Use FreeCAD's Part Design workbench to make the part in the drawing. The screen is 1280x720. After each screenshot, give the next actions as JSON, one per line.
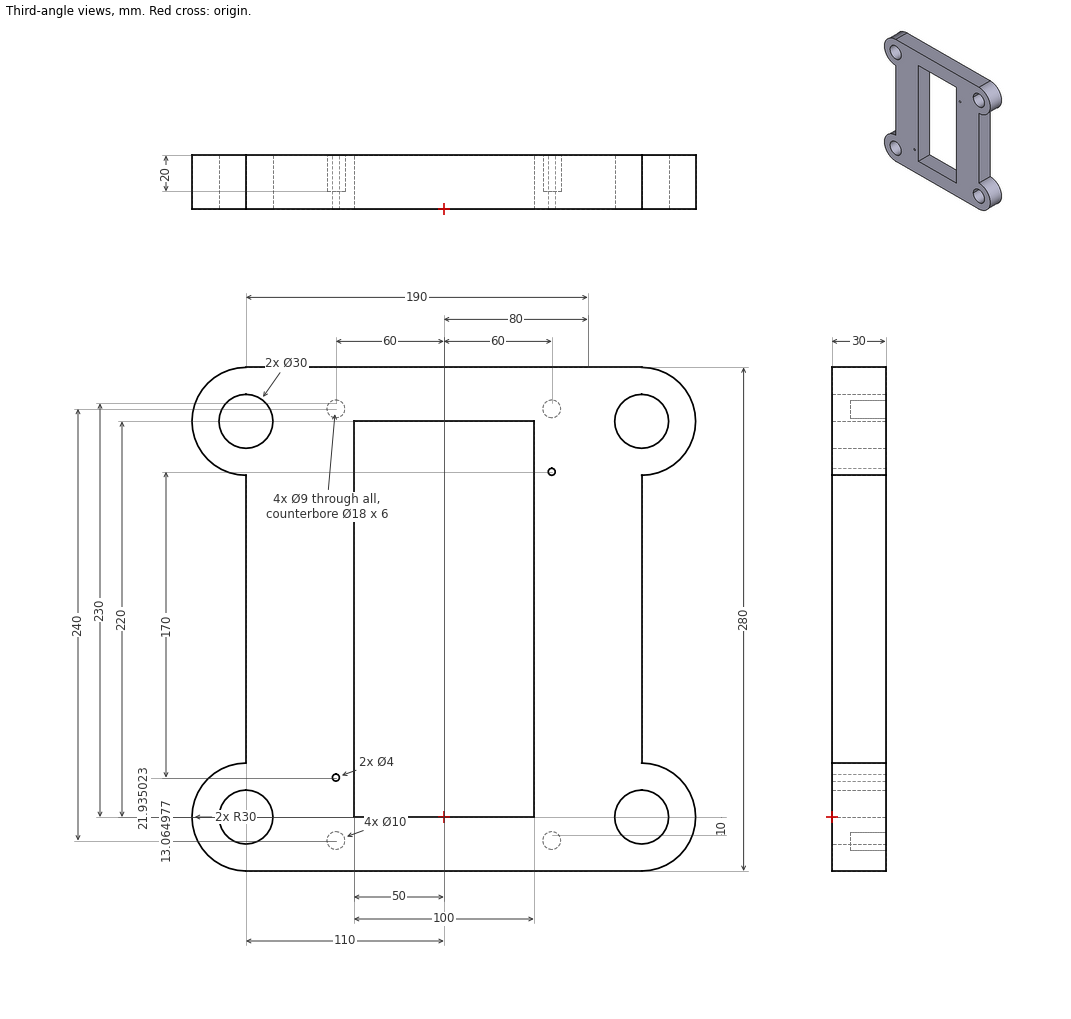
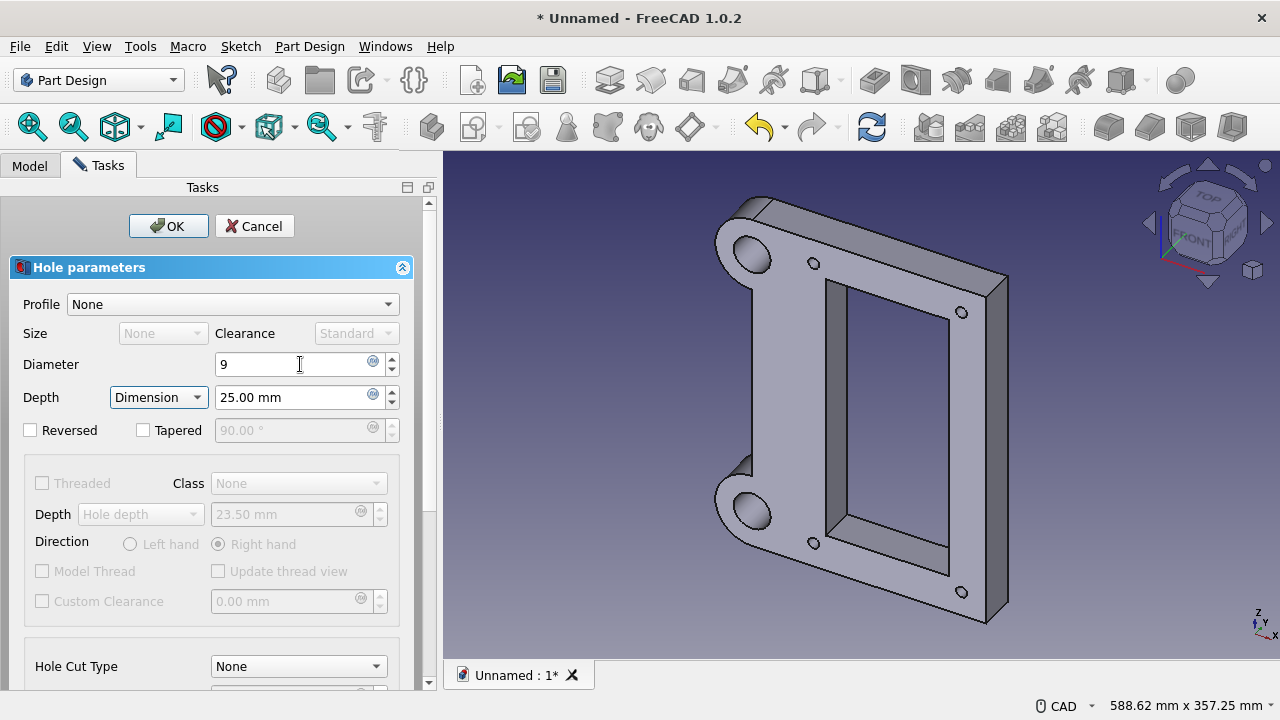
{"action": "left_click", "coordinate": [160, 398]}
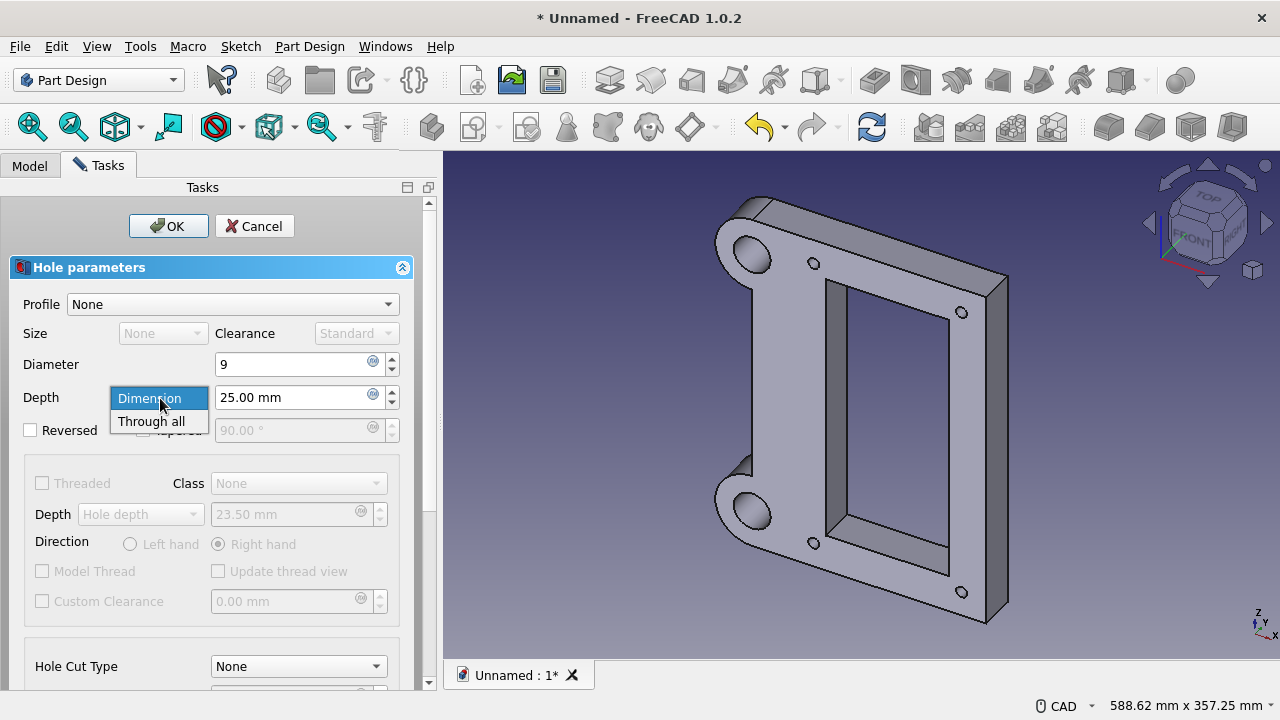
{"action": "left_click", "coordinate": [158, 422]}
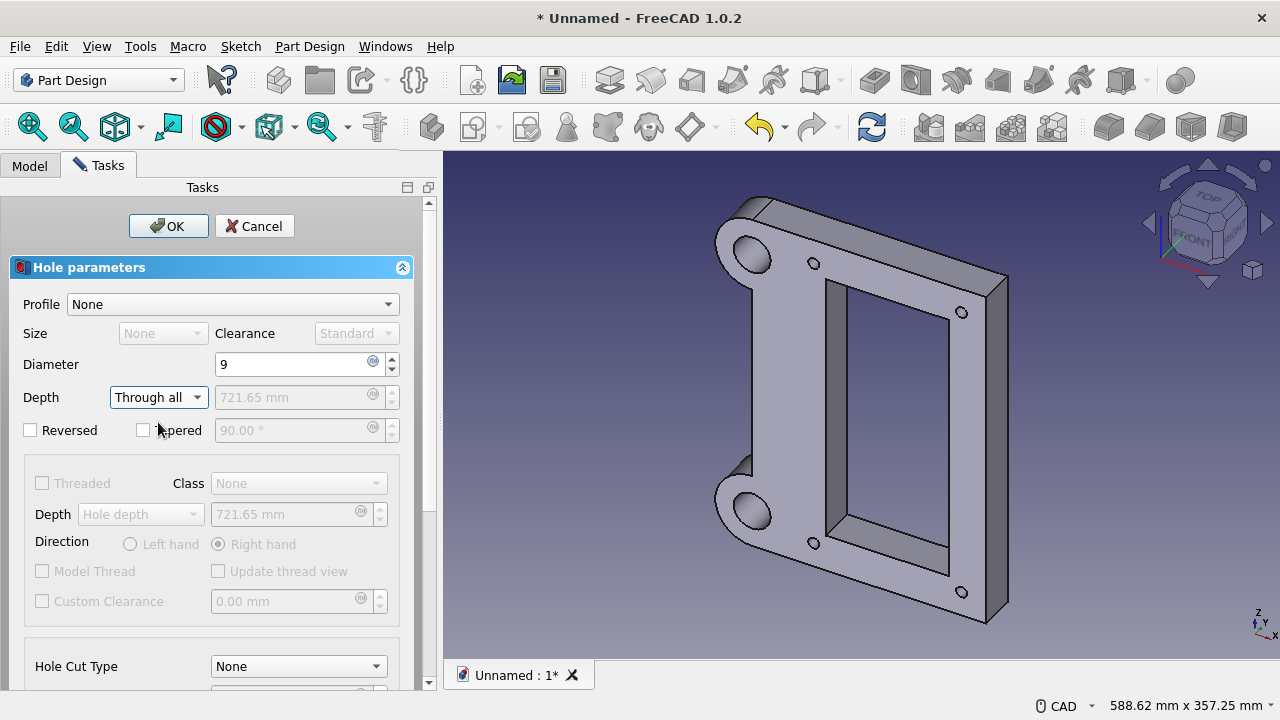
{"action": "left_click", "coordinate": [300, 666]}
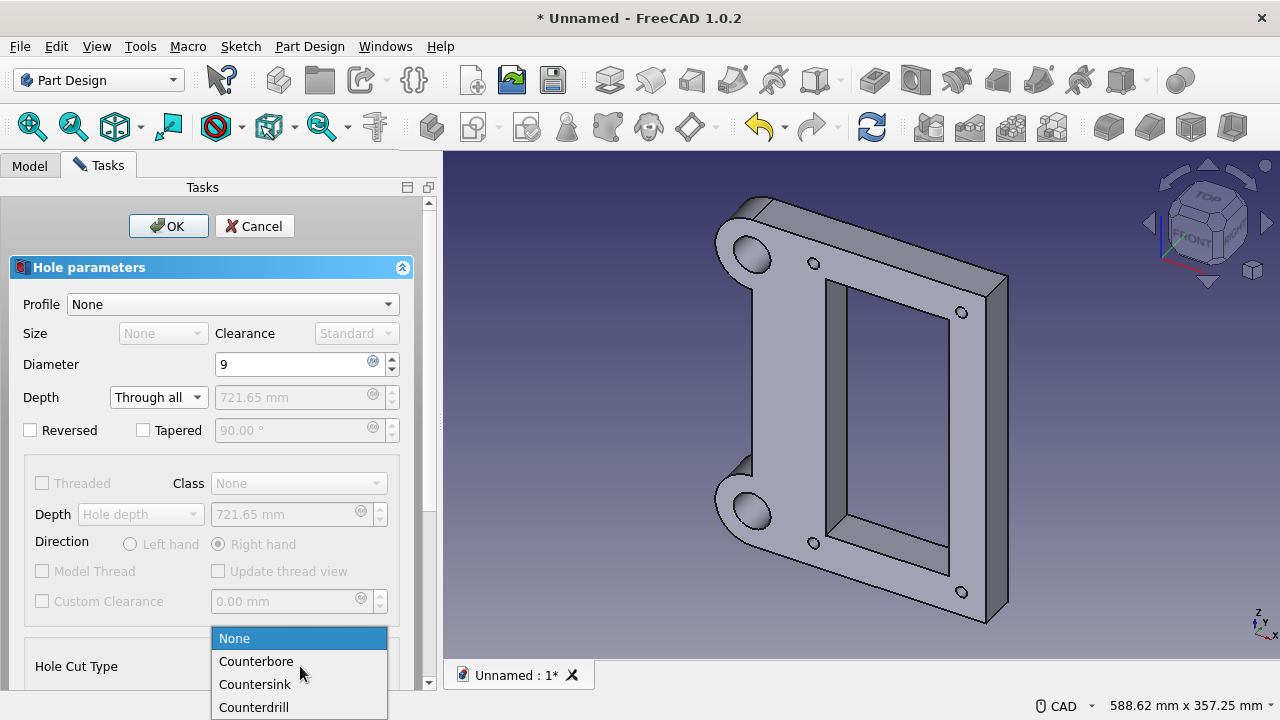
{"action": "left_click", "coordinate": [298, 662]}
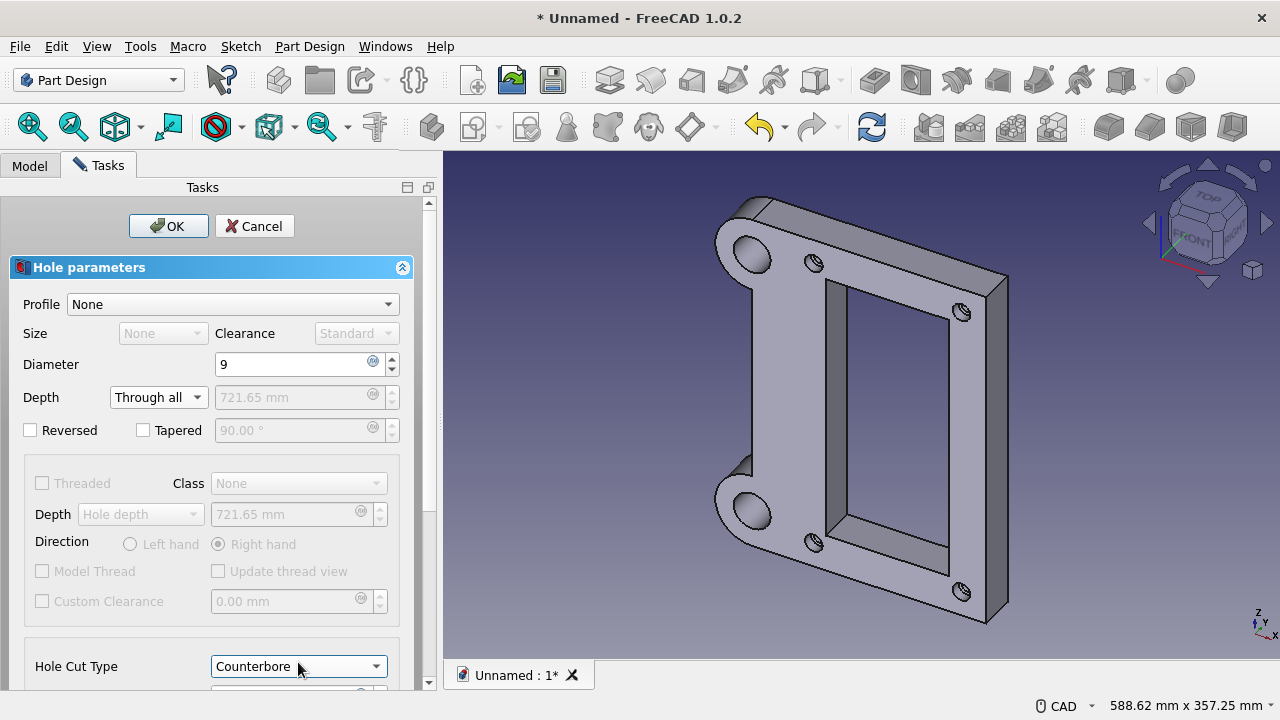
{"action": "scroll", "coordinate": [429, 444], "scroll_direction": "down", "scroll_amount": 2}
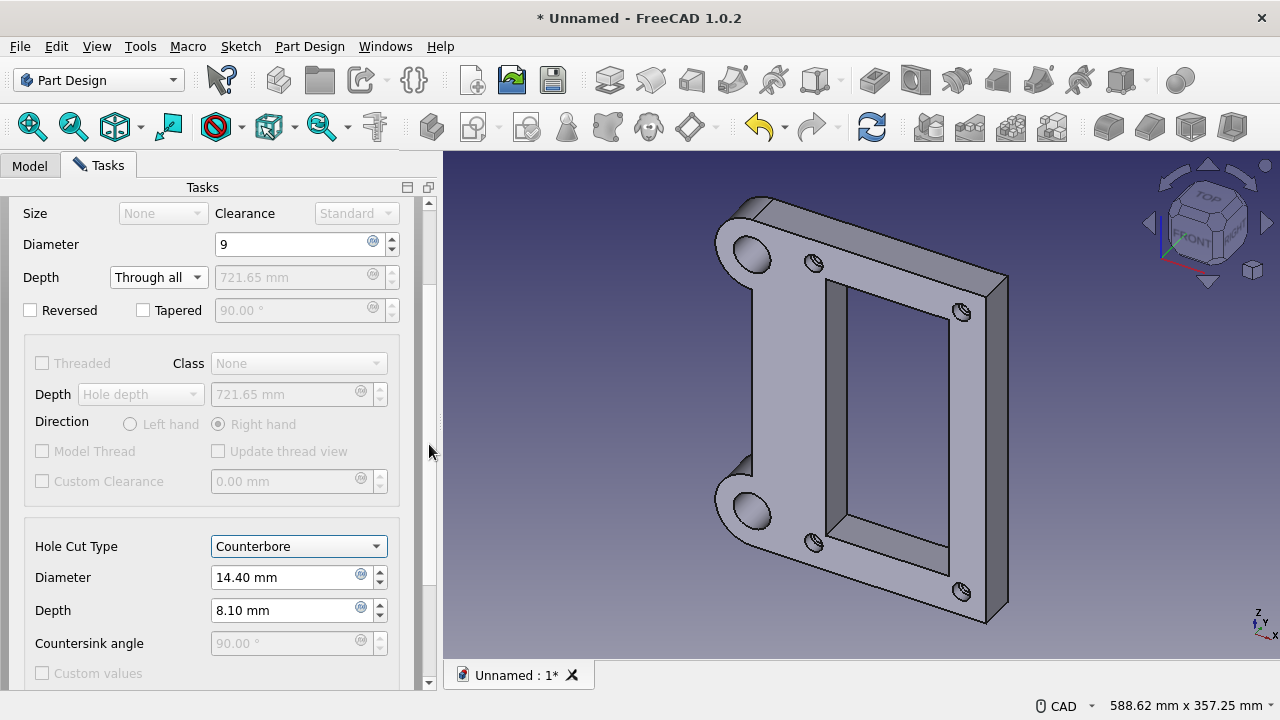
{"action": "triple_click", "coordinate": [292, 578]}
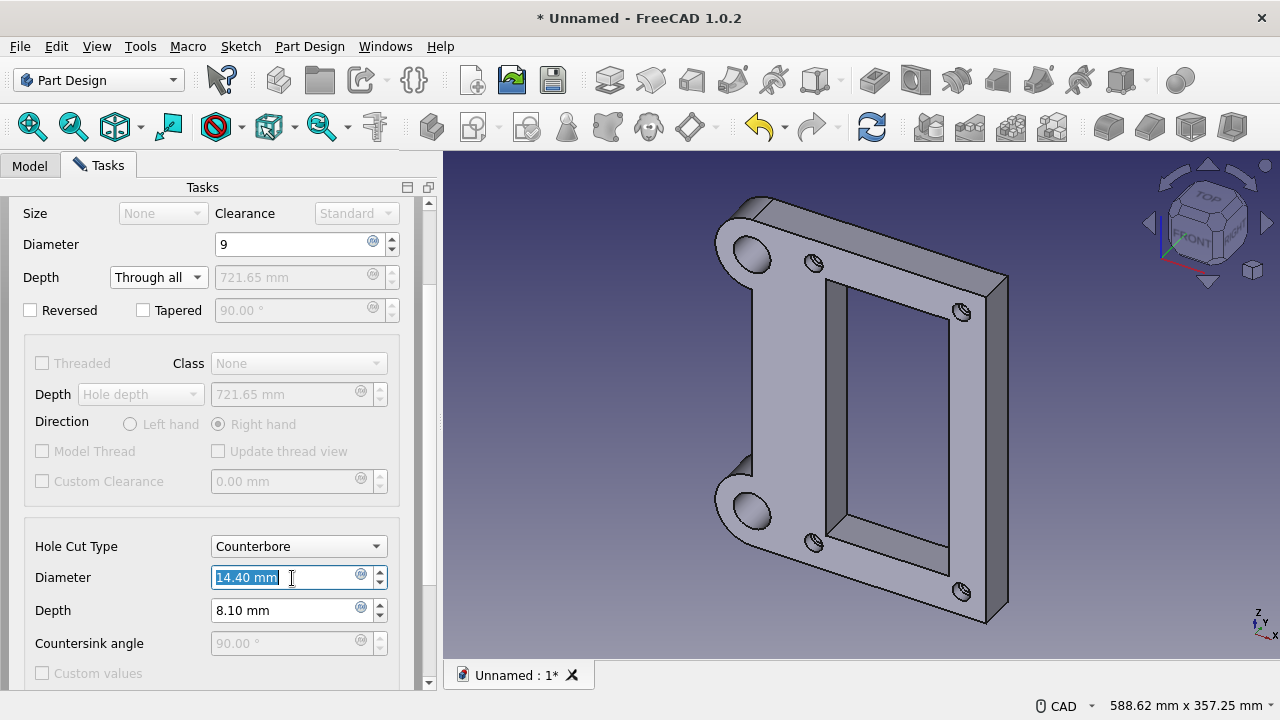
{"action": "type", "text": "18"}
{"action": "key", "text": "Tab"}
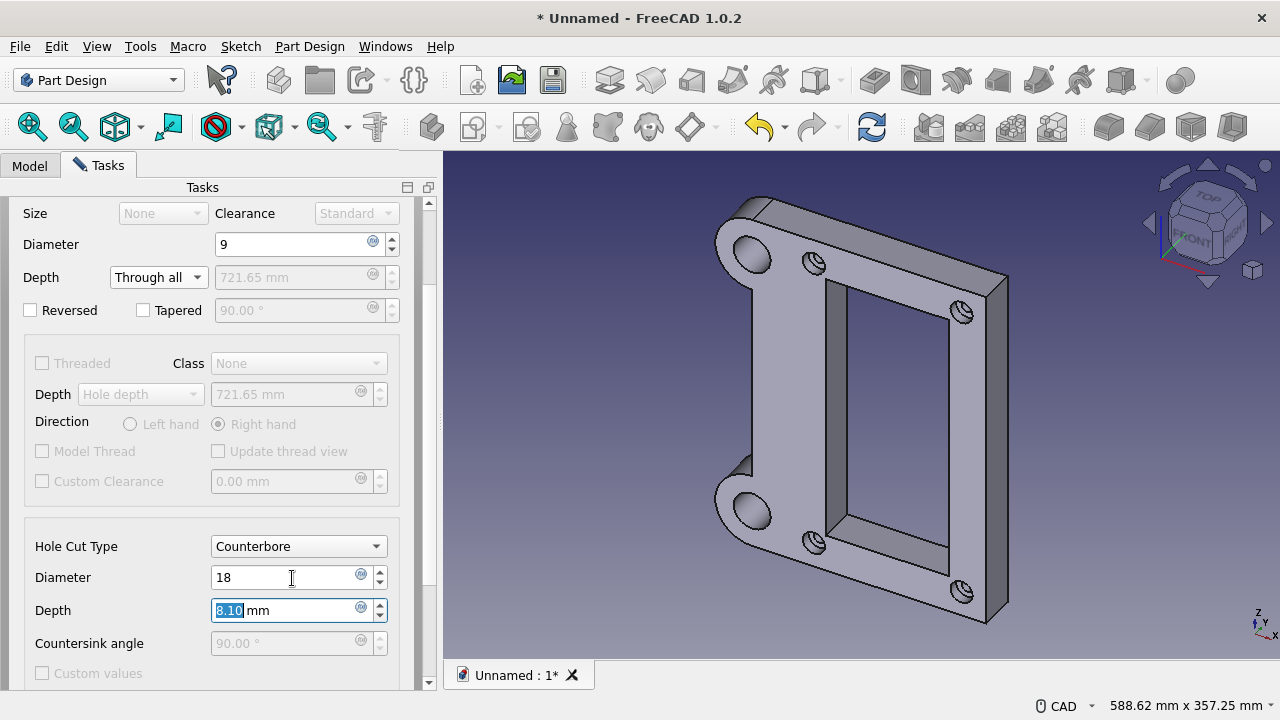
{"action": "type", "text": "6"}
{"action": "key", "text": "Tab"}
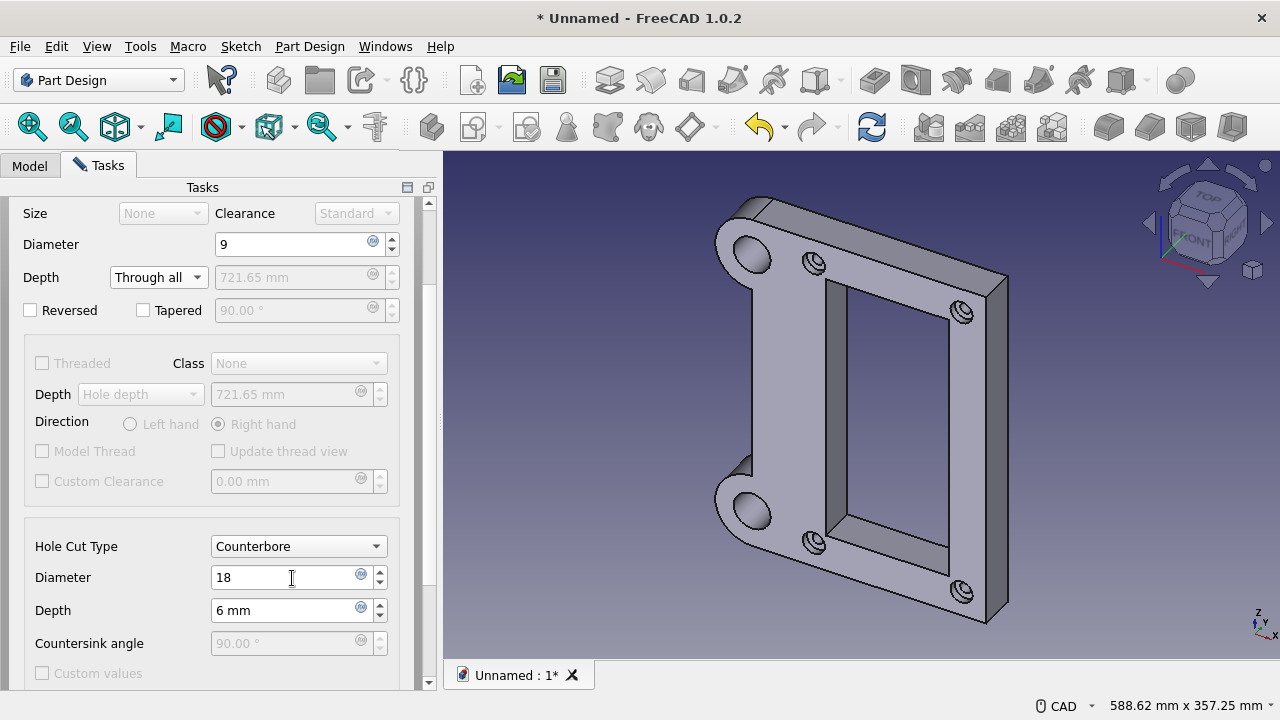
{"action": "scroll", "coordinate": [429, 444], "scroll_direction": "up", "scroll_amount": 3}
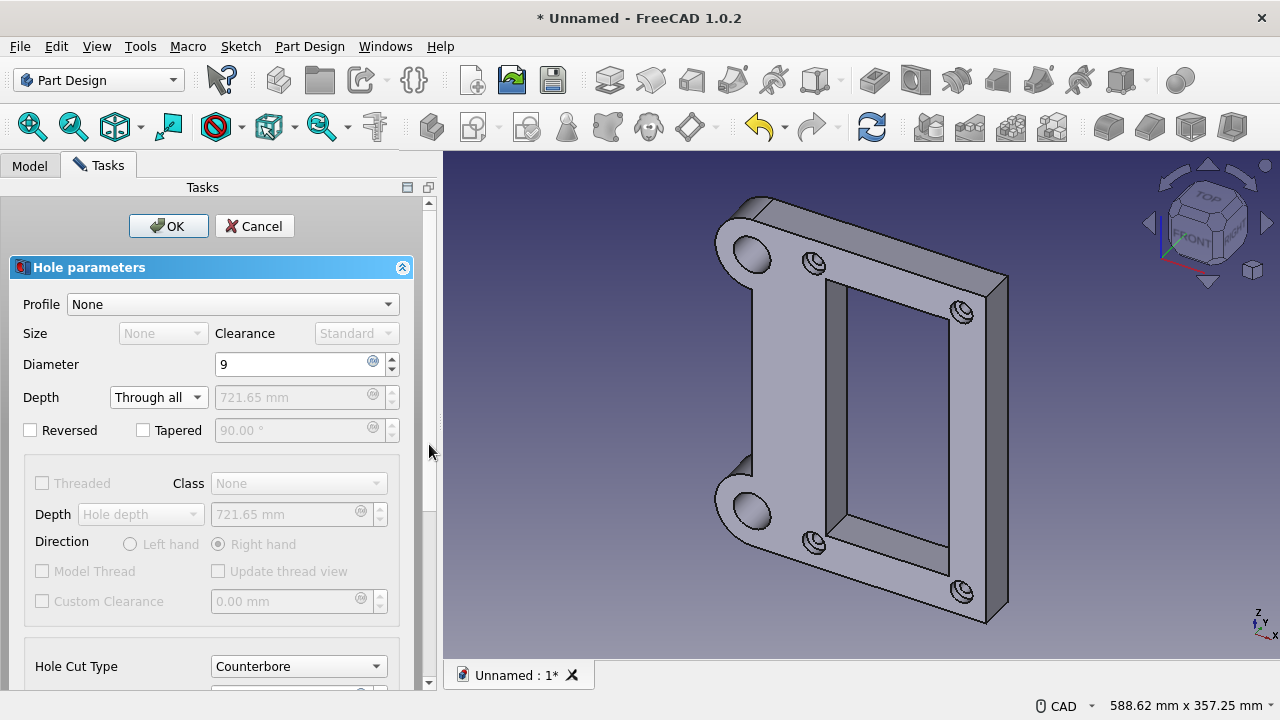
{"action": "left_click", "coordinate": [169, 226]}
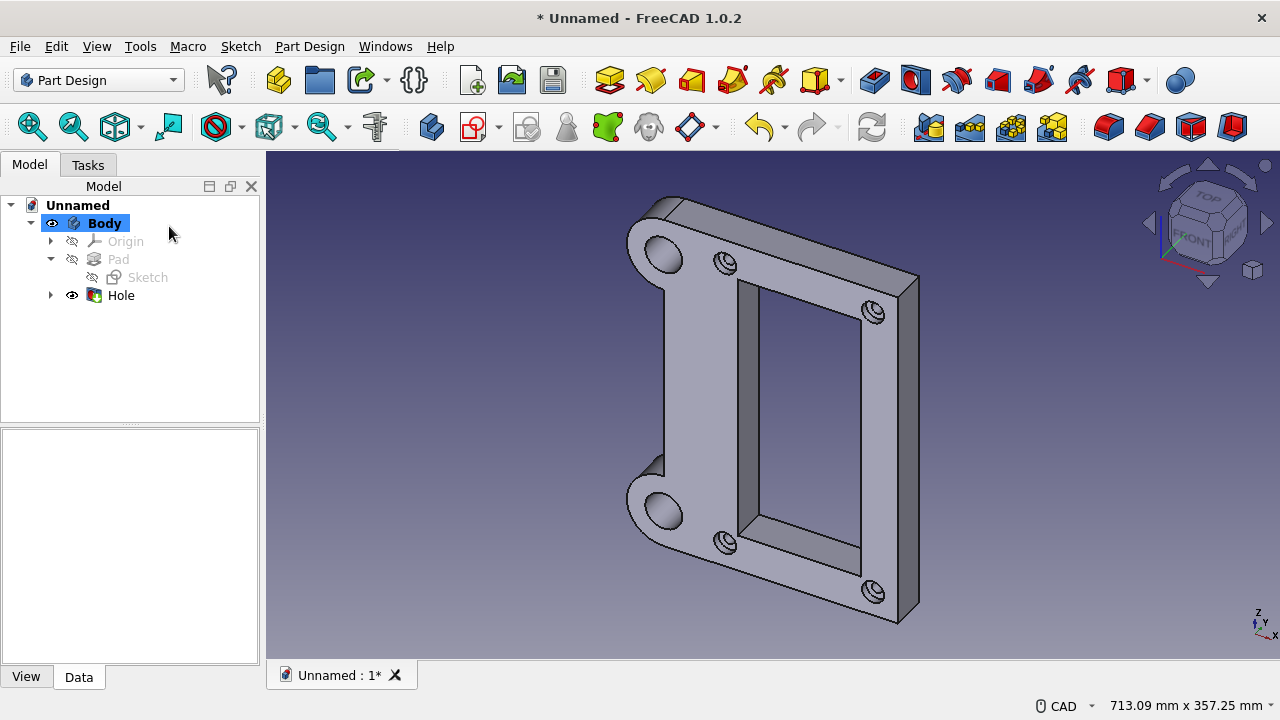
{"action": "left_click", "coordinate": [117, 259]}